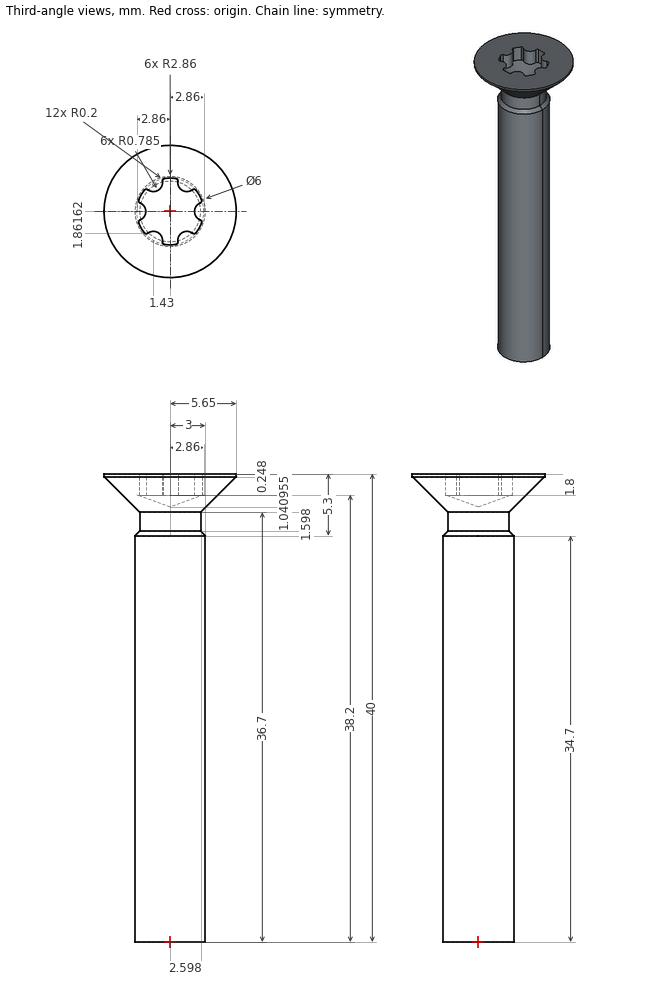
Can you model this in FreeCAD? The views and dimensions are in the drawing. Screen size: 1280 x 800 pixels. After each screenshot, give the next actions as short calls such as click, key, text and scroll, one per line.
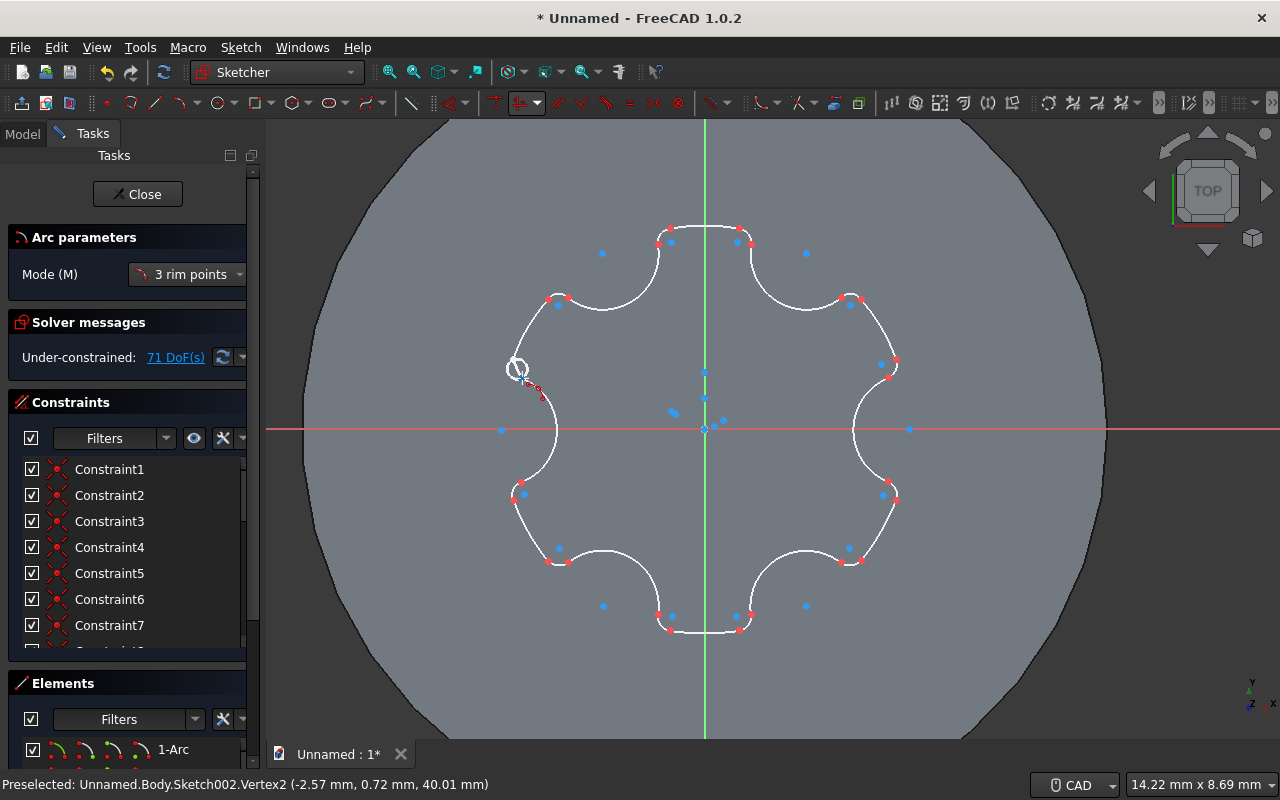
scroll(513, 370, up, 7)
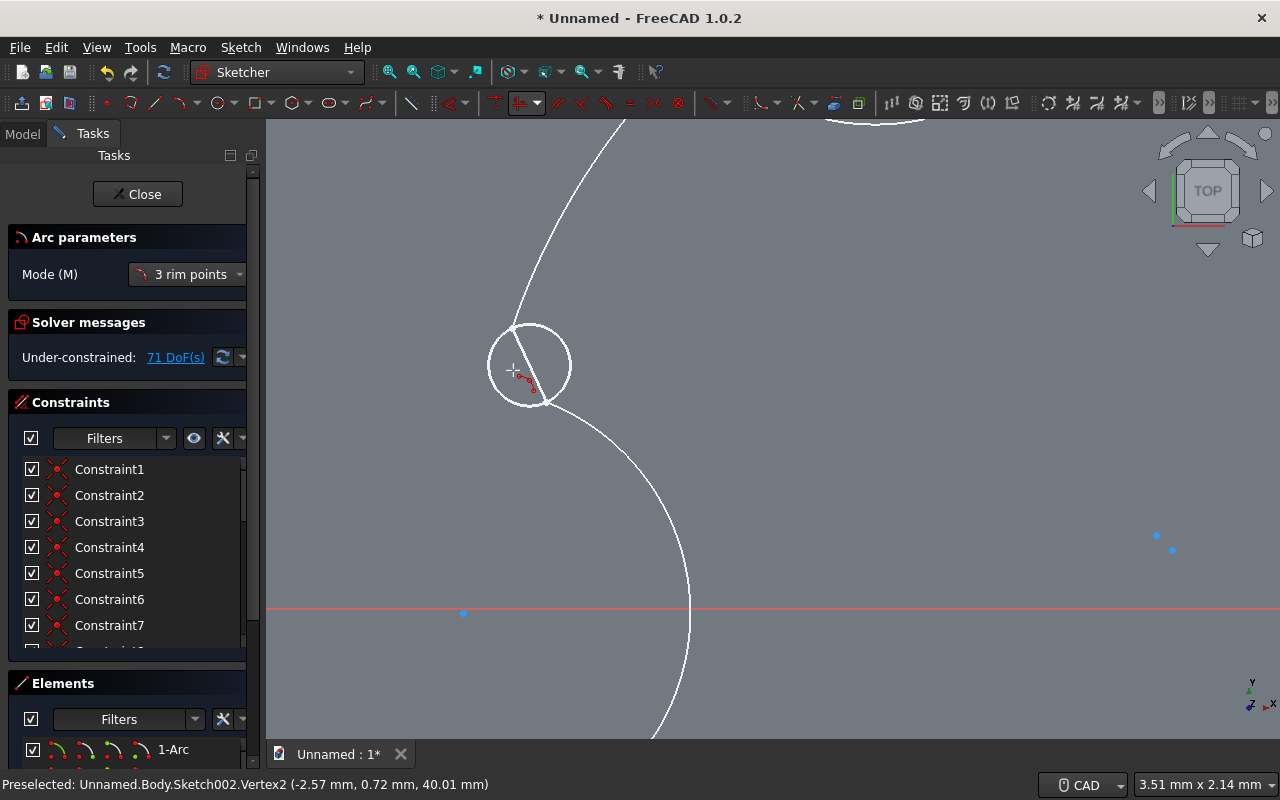
click(514, 368)
key(Escape)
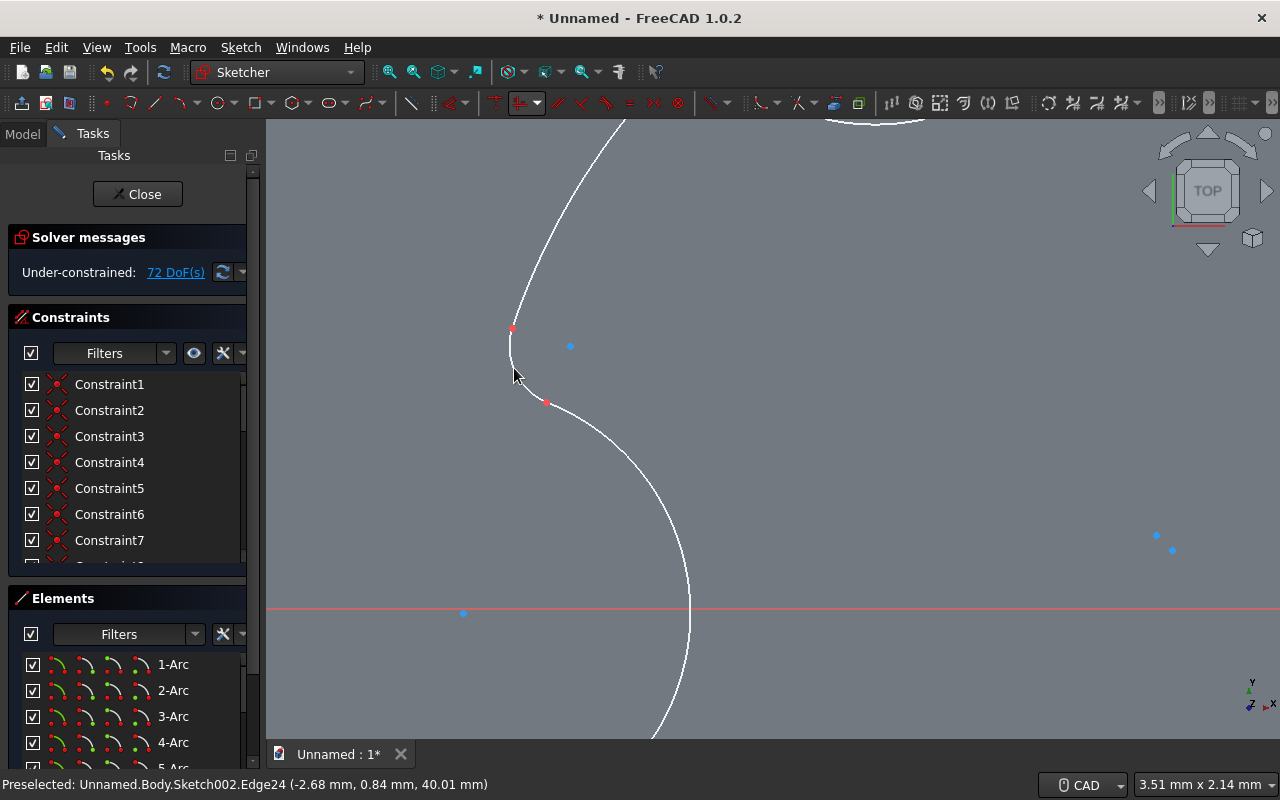
scroll(513, 370, down, 7)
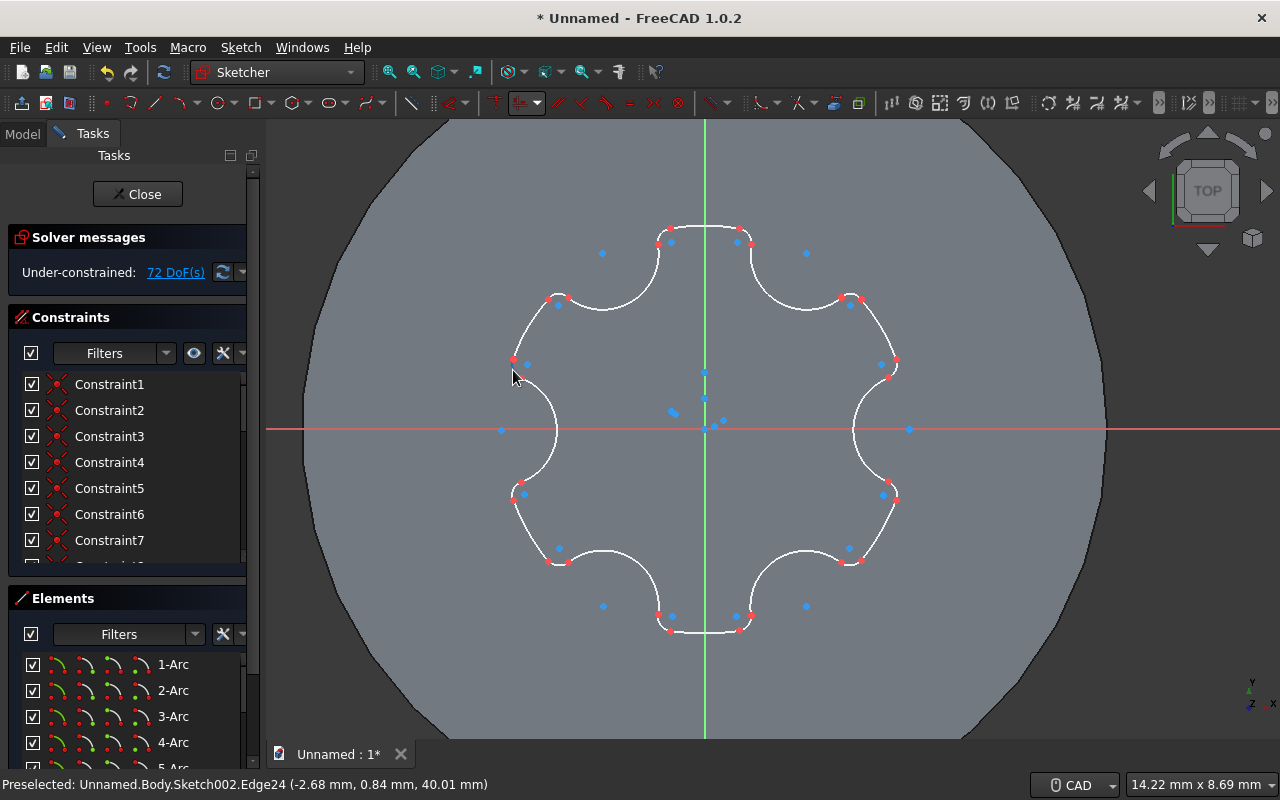
click(551, 405)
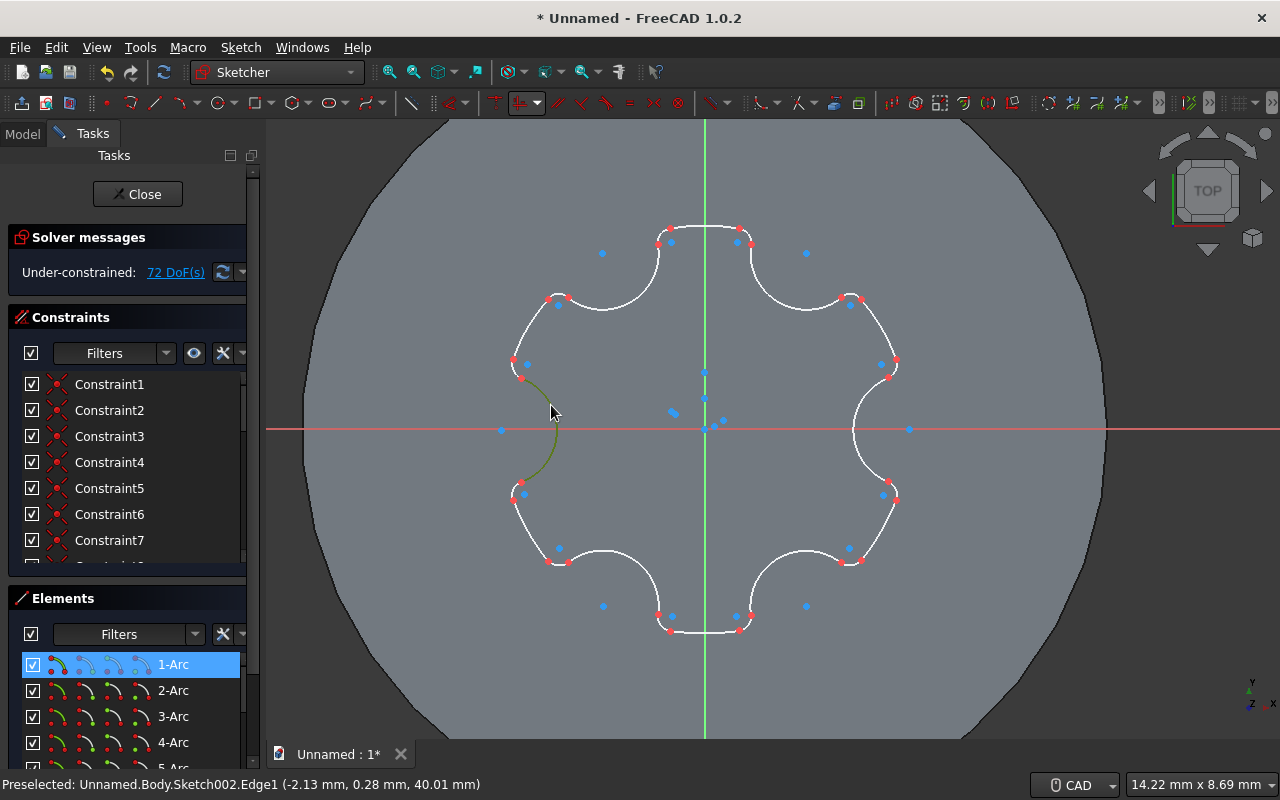
scroll(513, 489, up, 2)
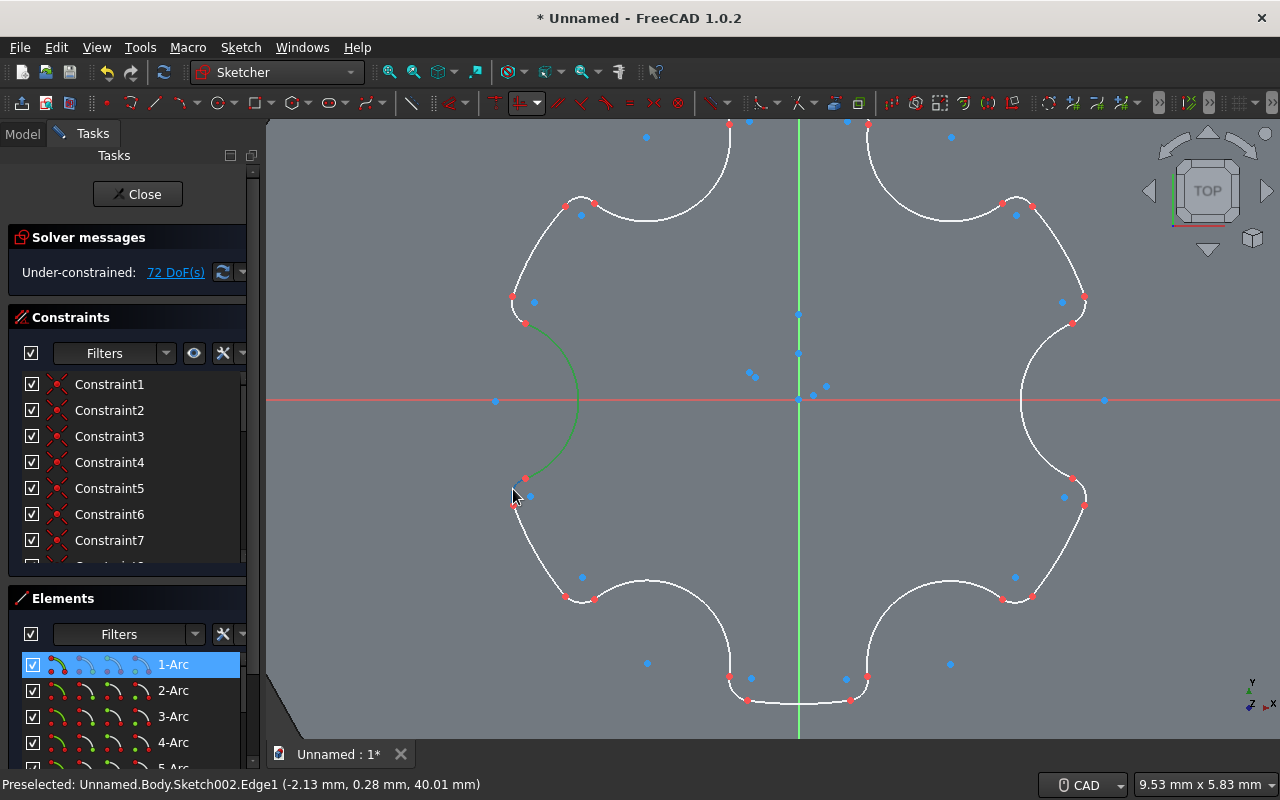
click(513, 489)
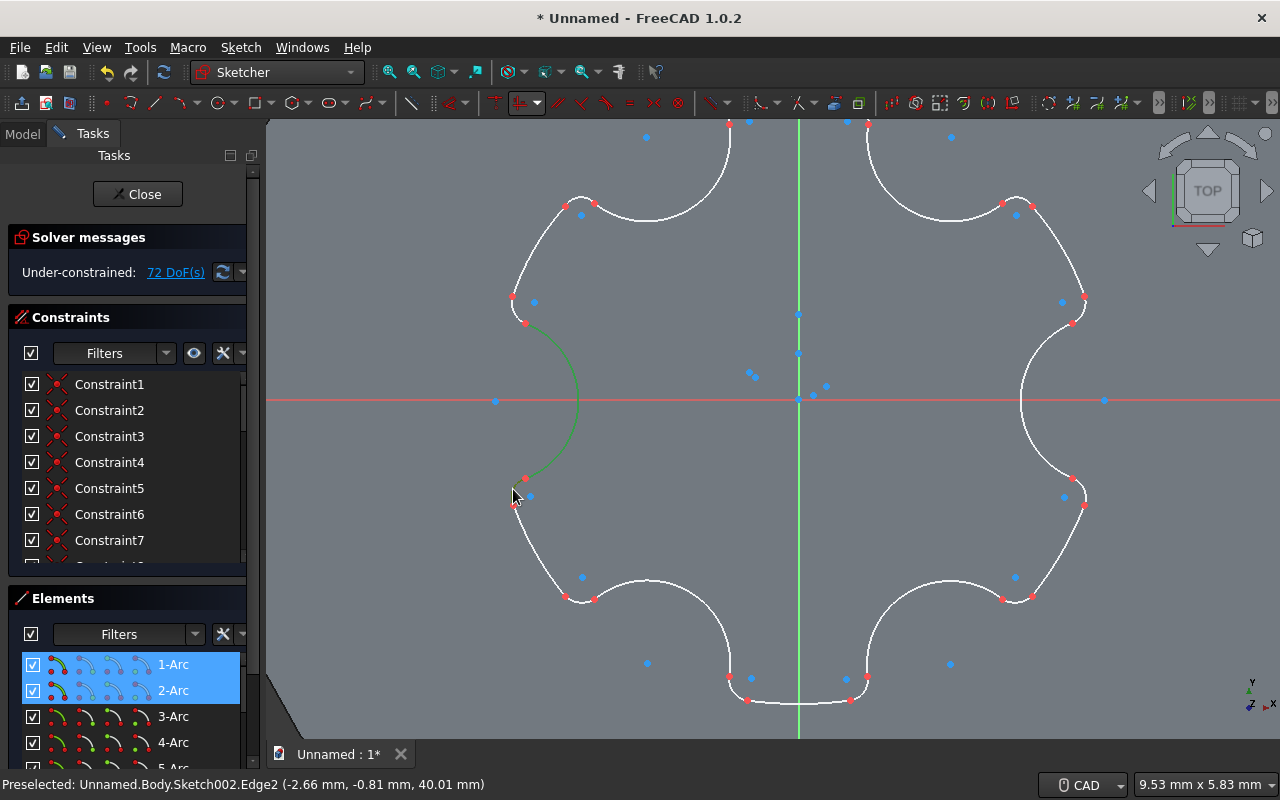
click(606, 104)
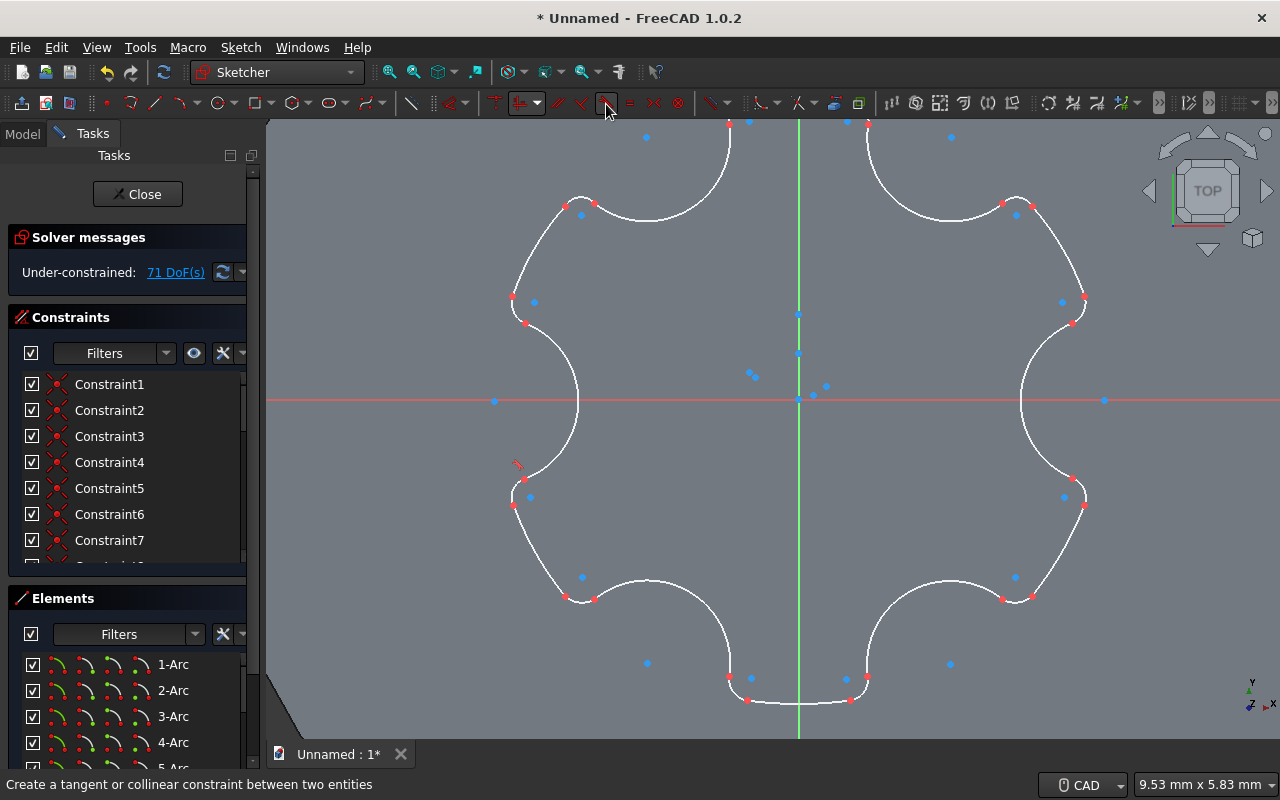
click(568, 440)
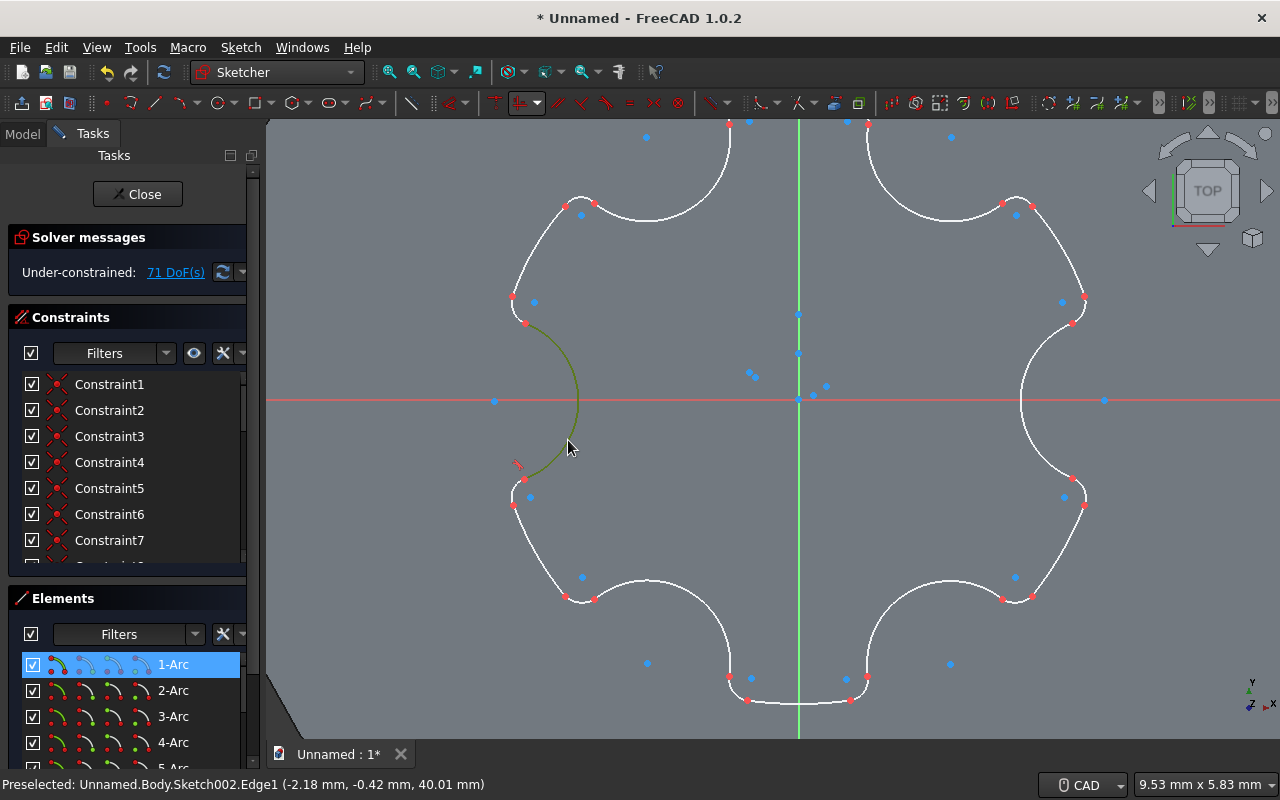
scroll(512, 306, up, 2)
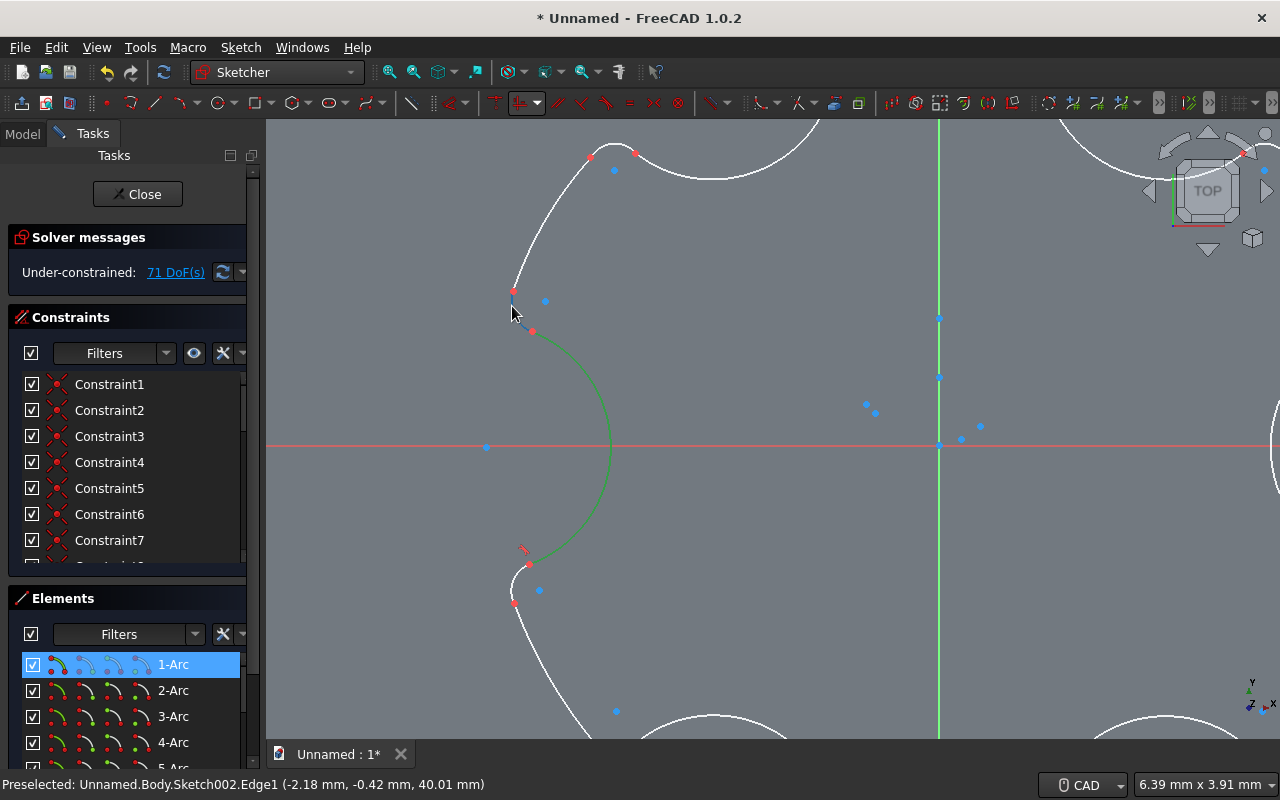
click(512, 306)